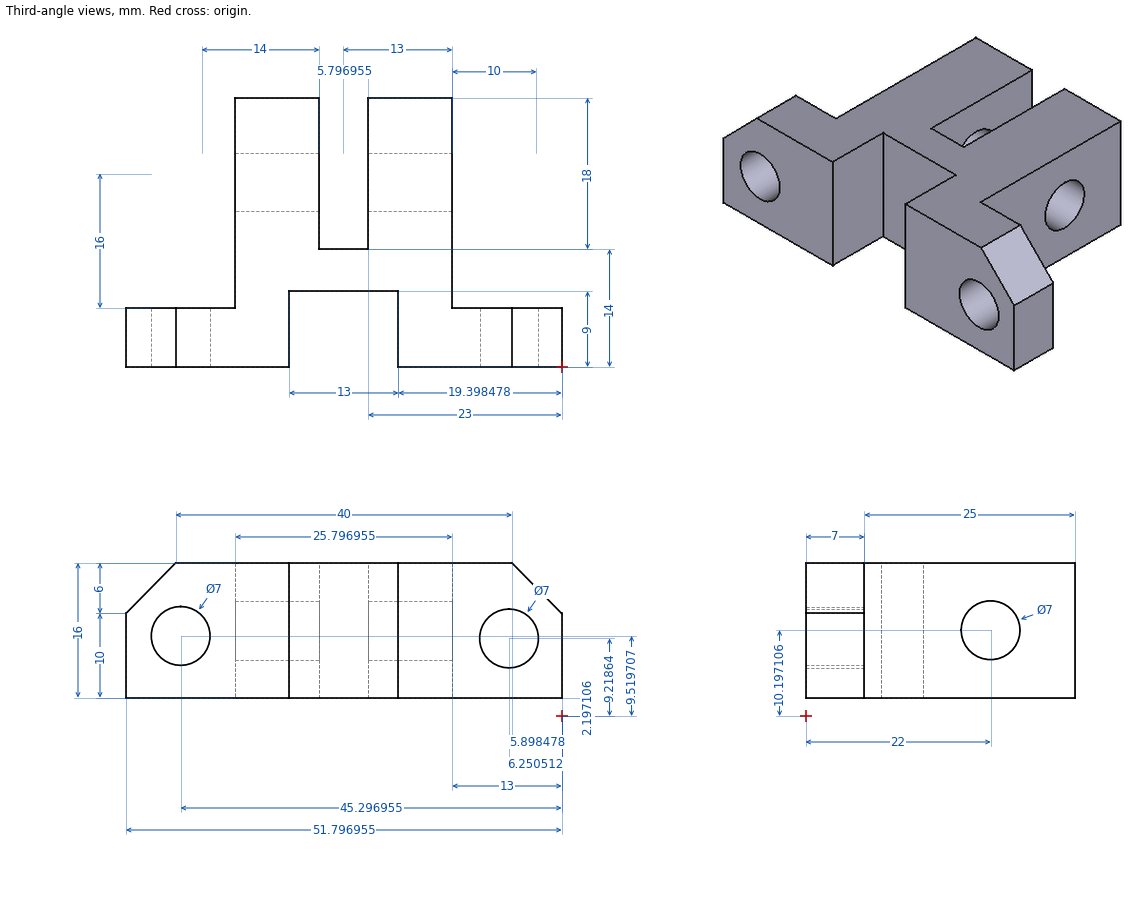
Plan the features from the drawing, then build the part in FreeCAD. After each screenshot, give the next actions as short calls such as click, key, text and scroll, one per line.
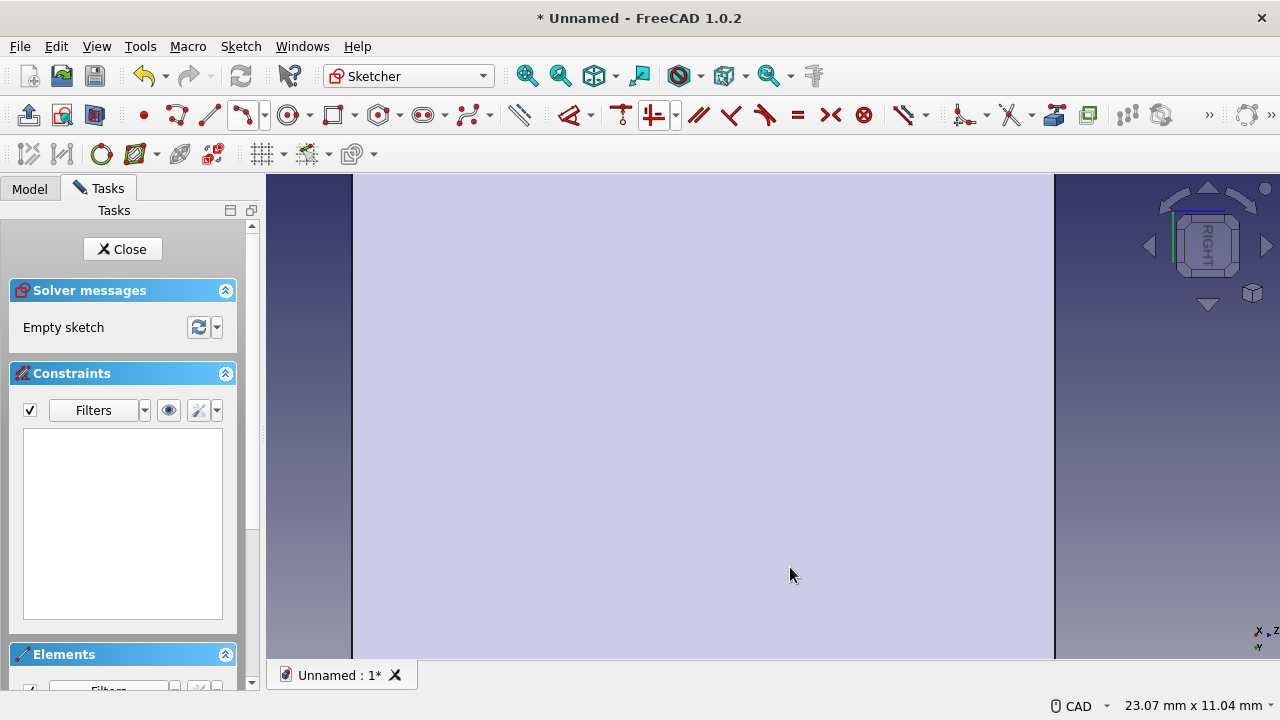
click(288, 116)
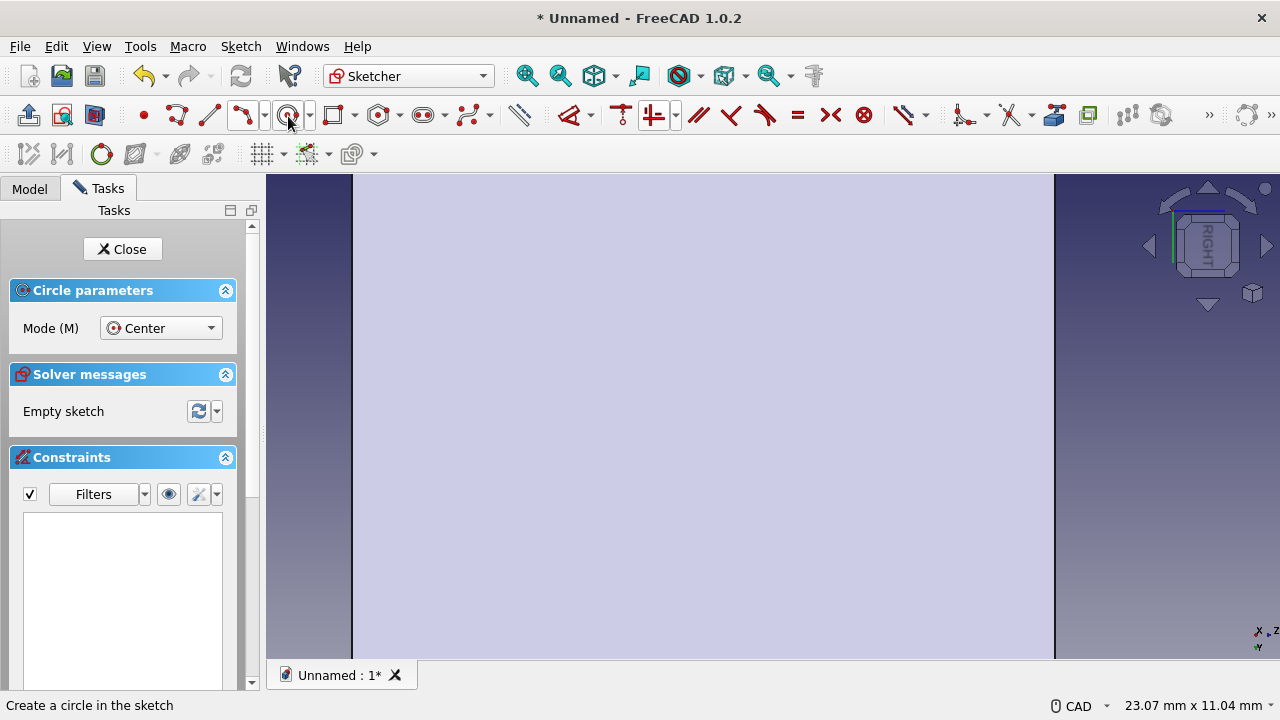
click(704, 412)
click(813, 303)
key(Escape)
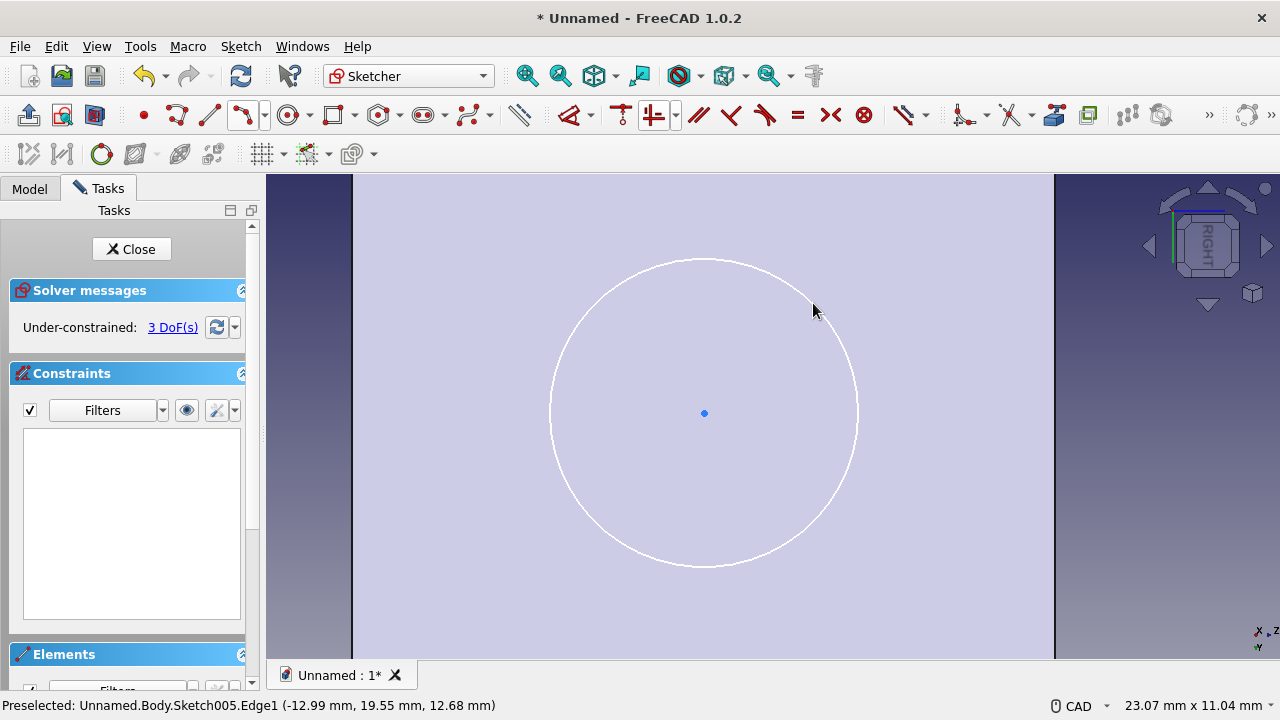
key(d)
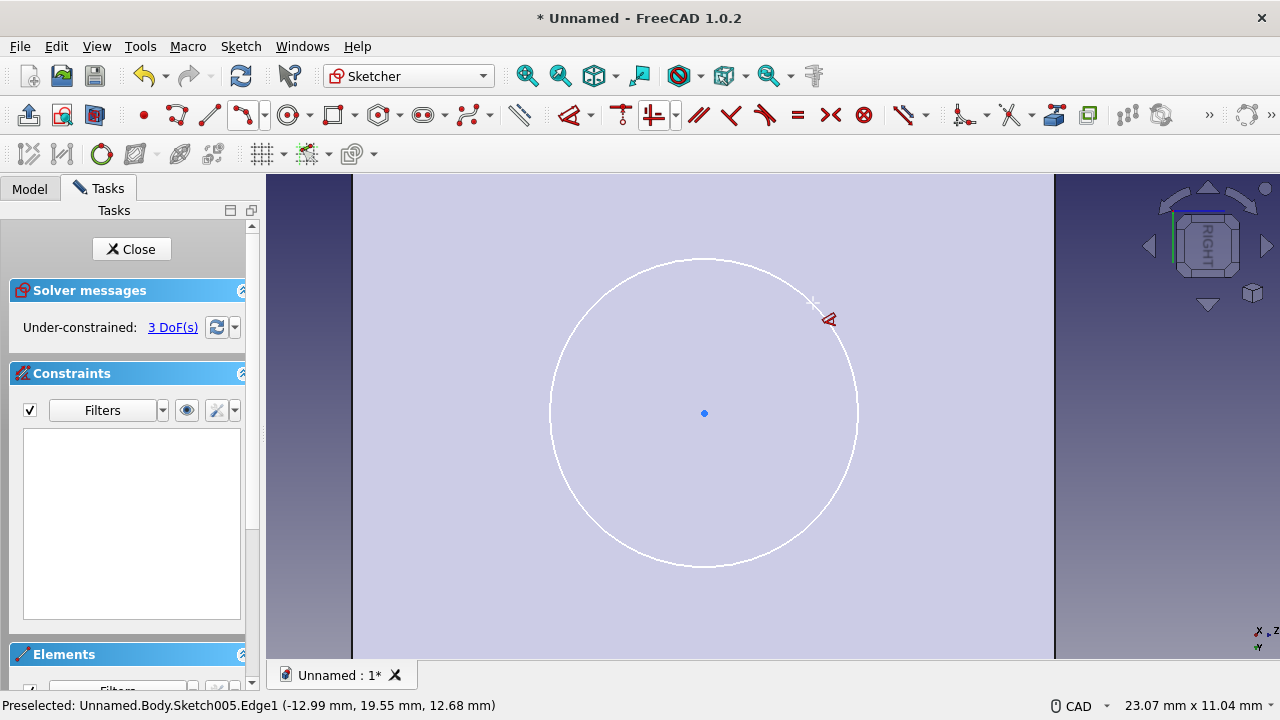
click(813, 304)
click(836, 281)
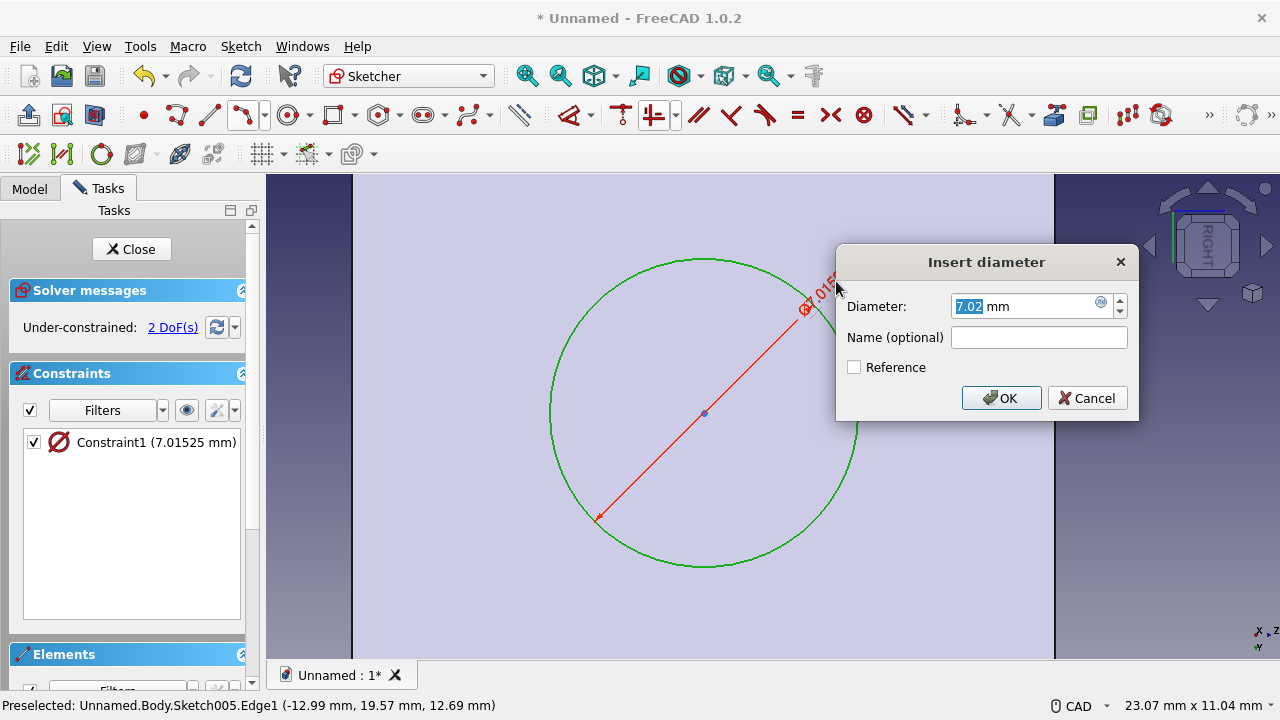
text(7)
key(Return)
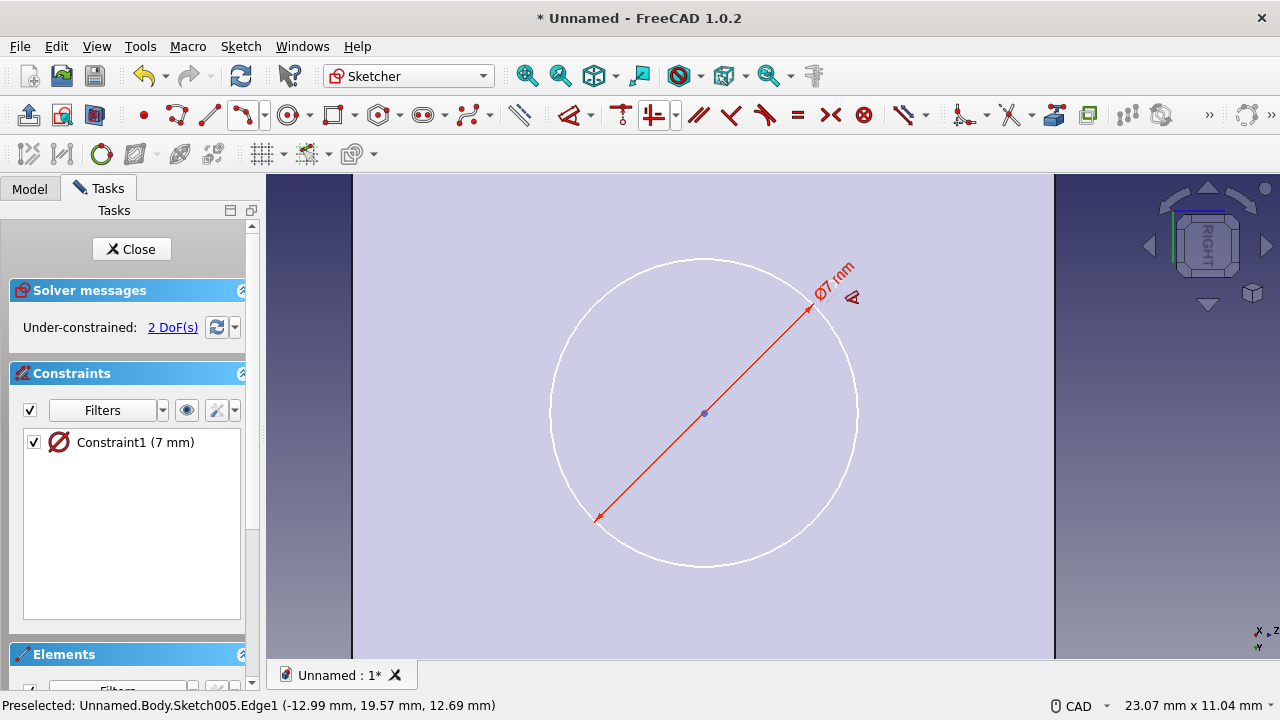
click(704, 413)
click(738, 308)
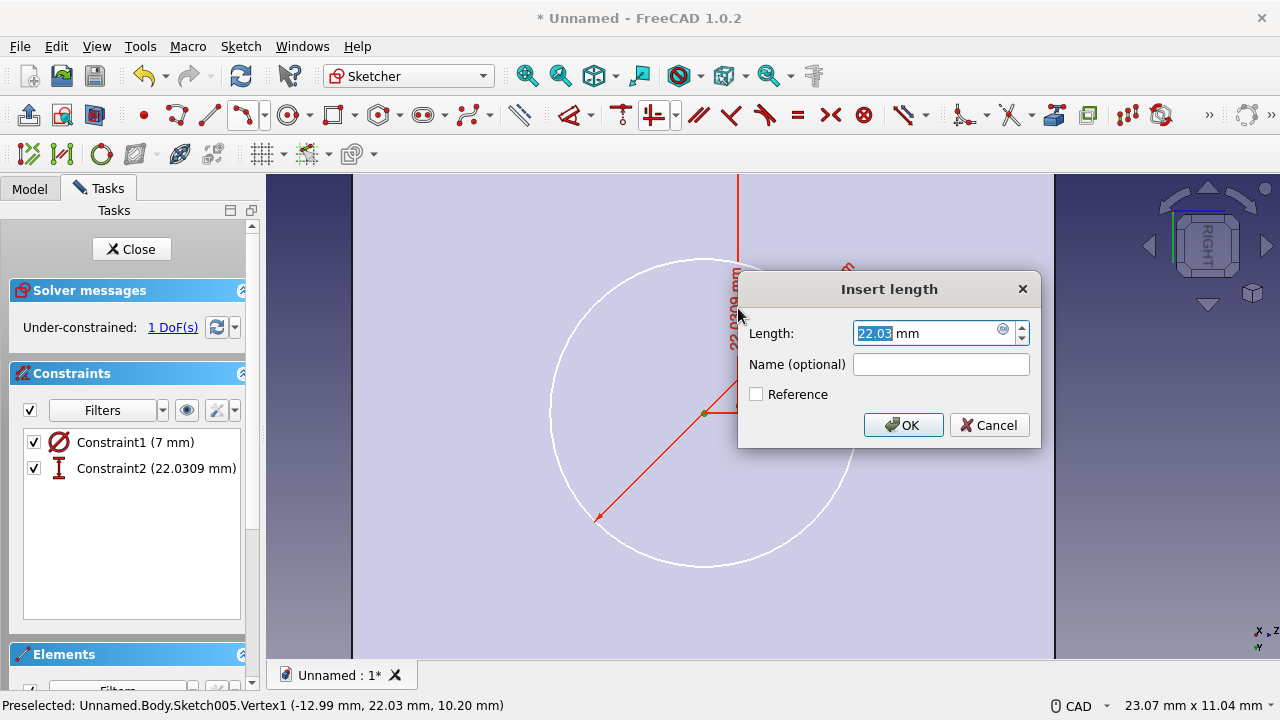
text(22)
key(Return)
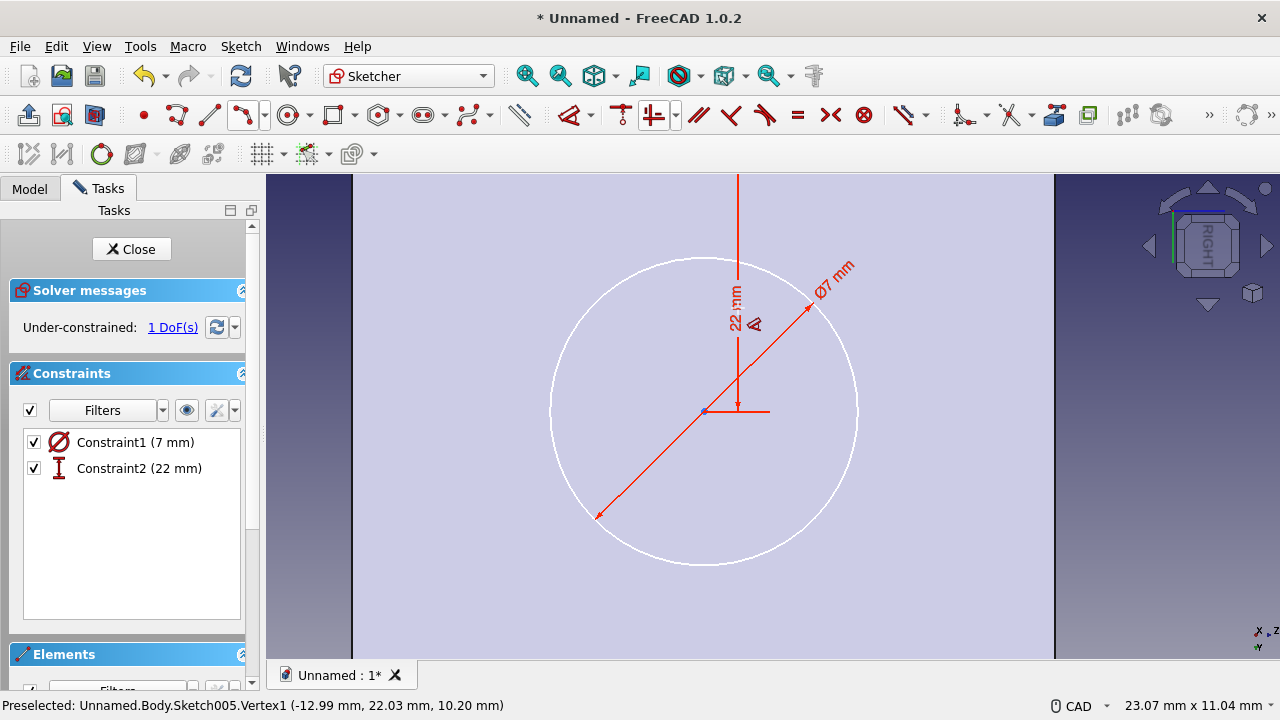
click(704, 412)
click(499, 446)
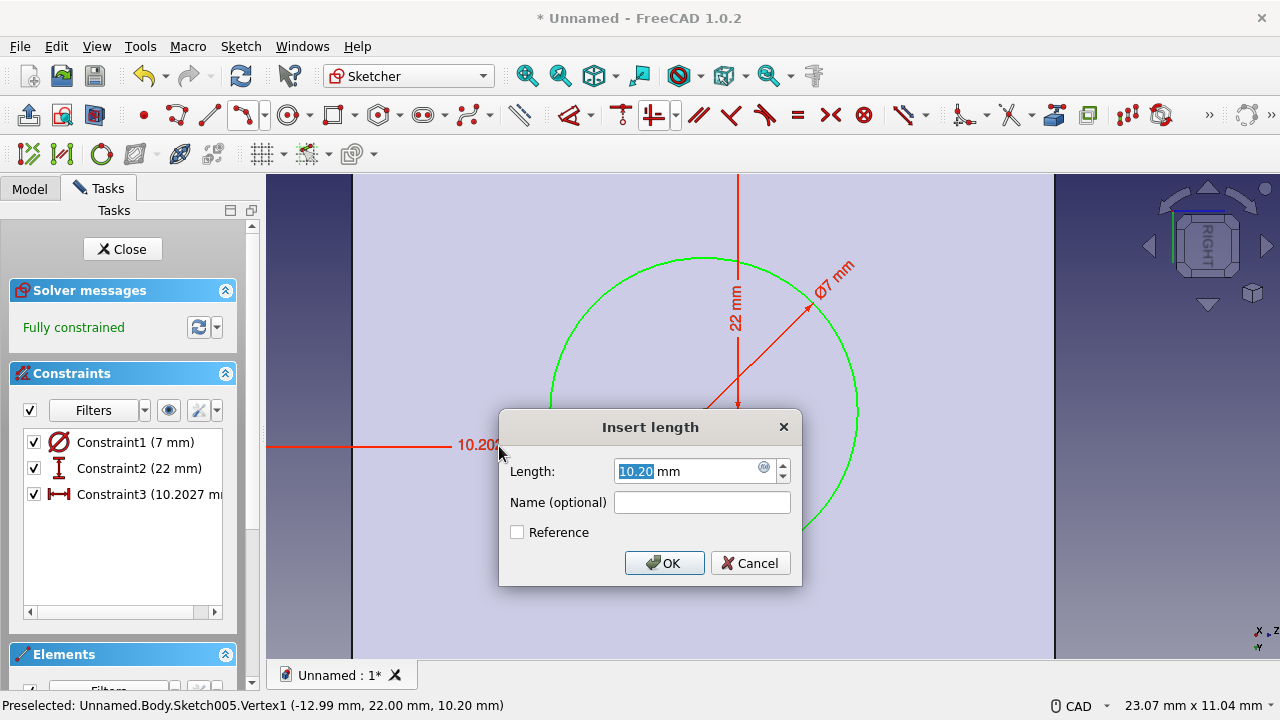
text(10.197106)
key(Return)
key(Escape)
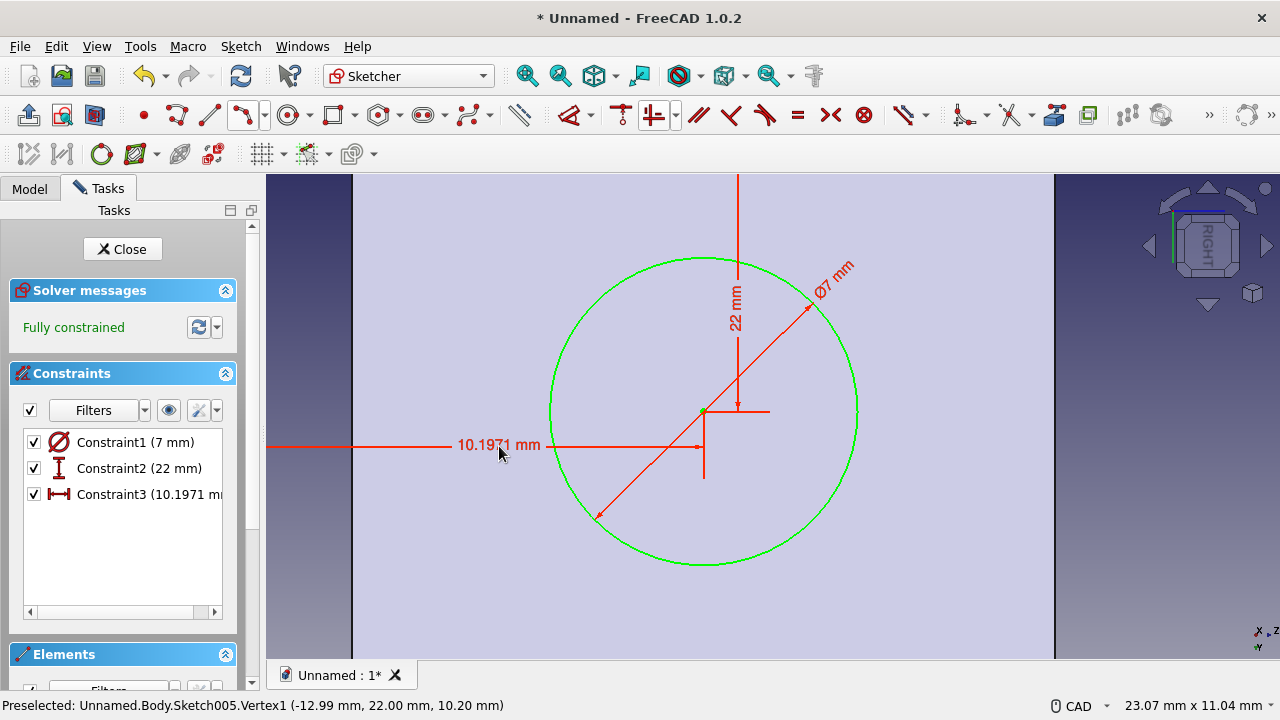
click(123, 249)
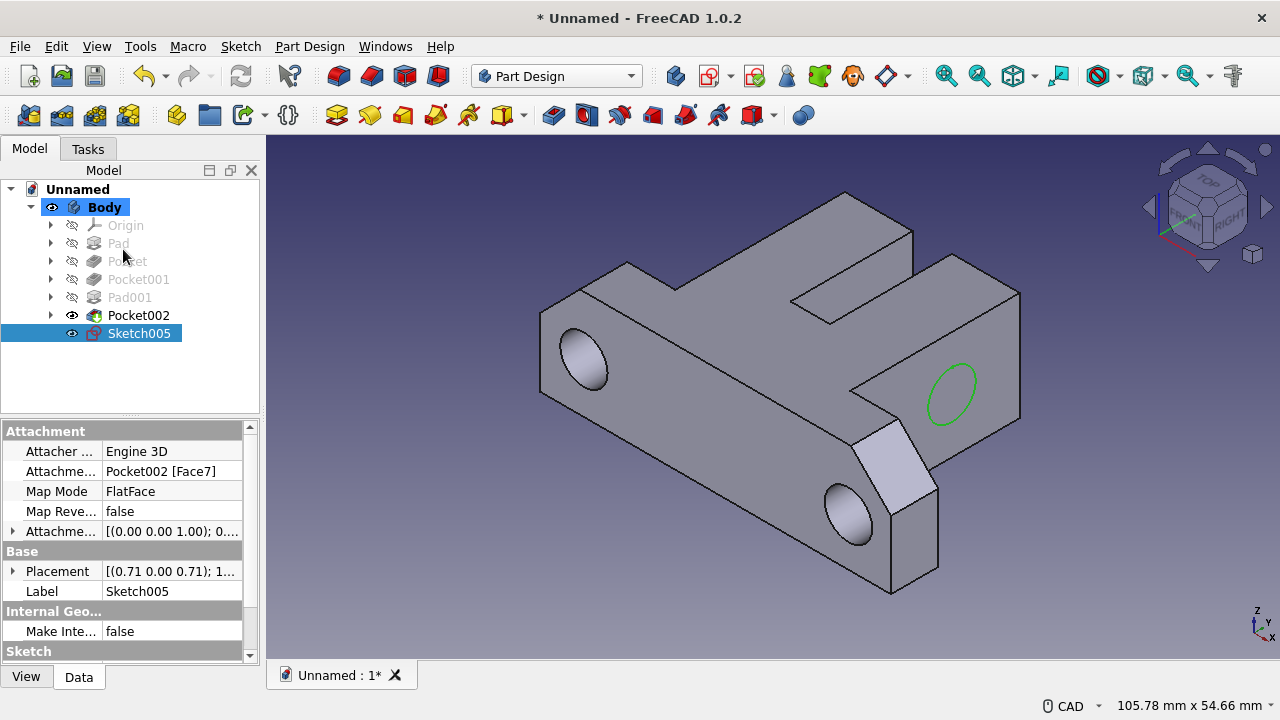
click(554, 116)